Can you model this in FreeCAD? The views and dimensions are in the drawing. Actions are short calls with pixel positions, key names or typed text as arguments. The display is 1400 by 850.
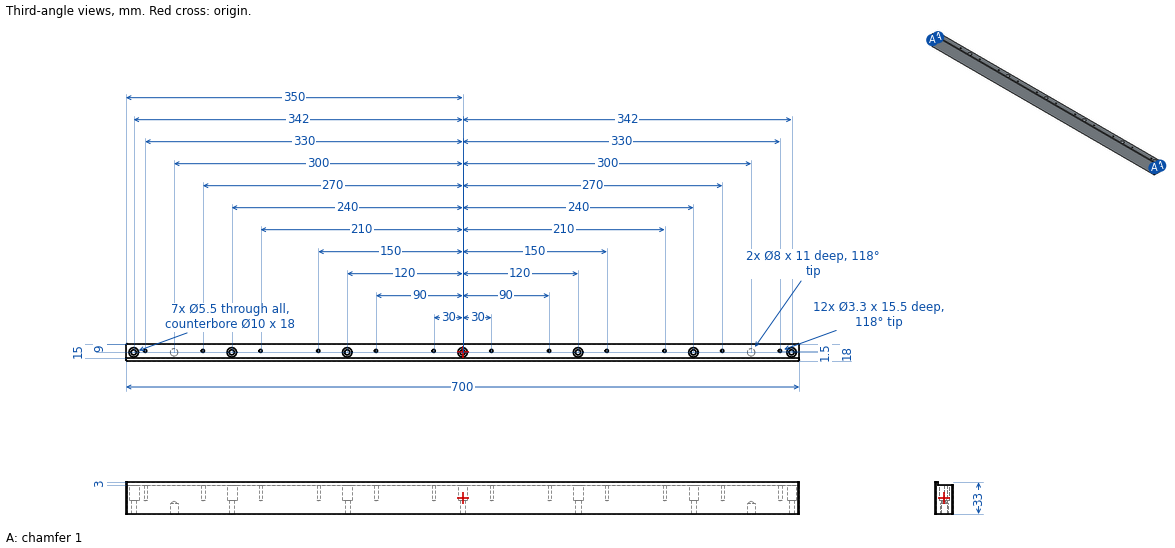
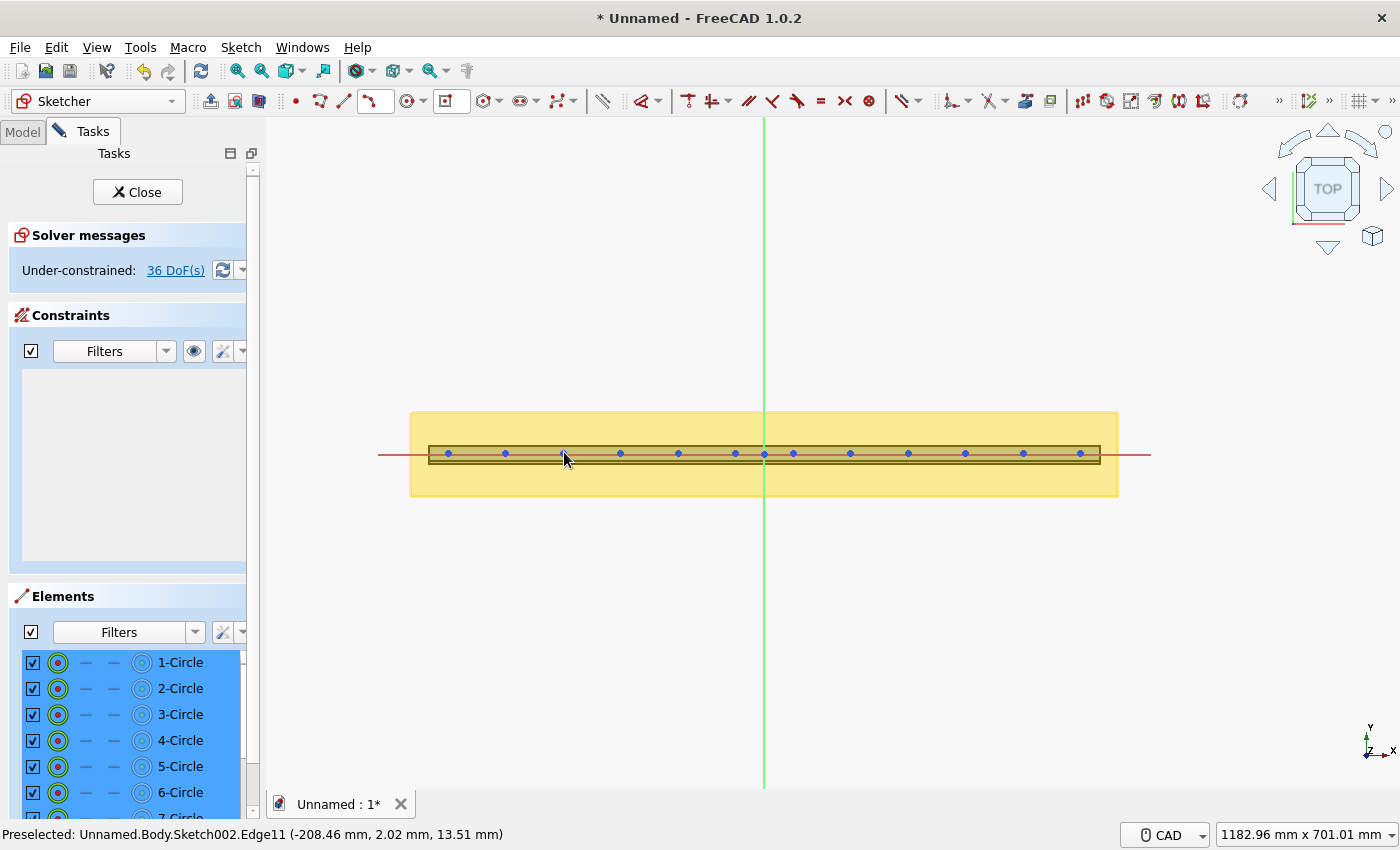
scroll(507, 452, up, 11)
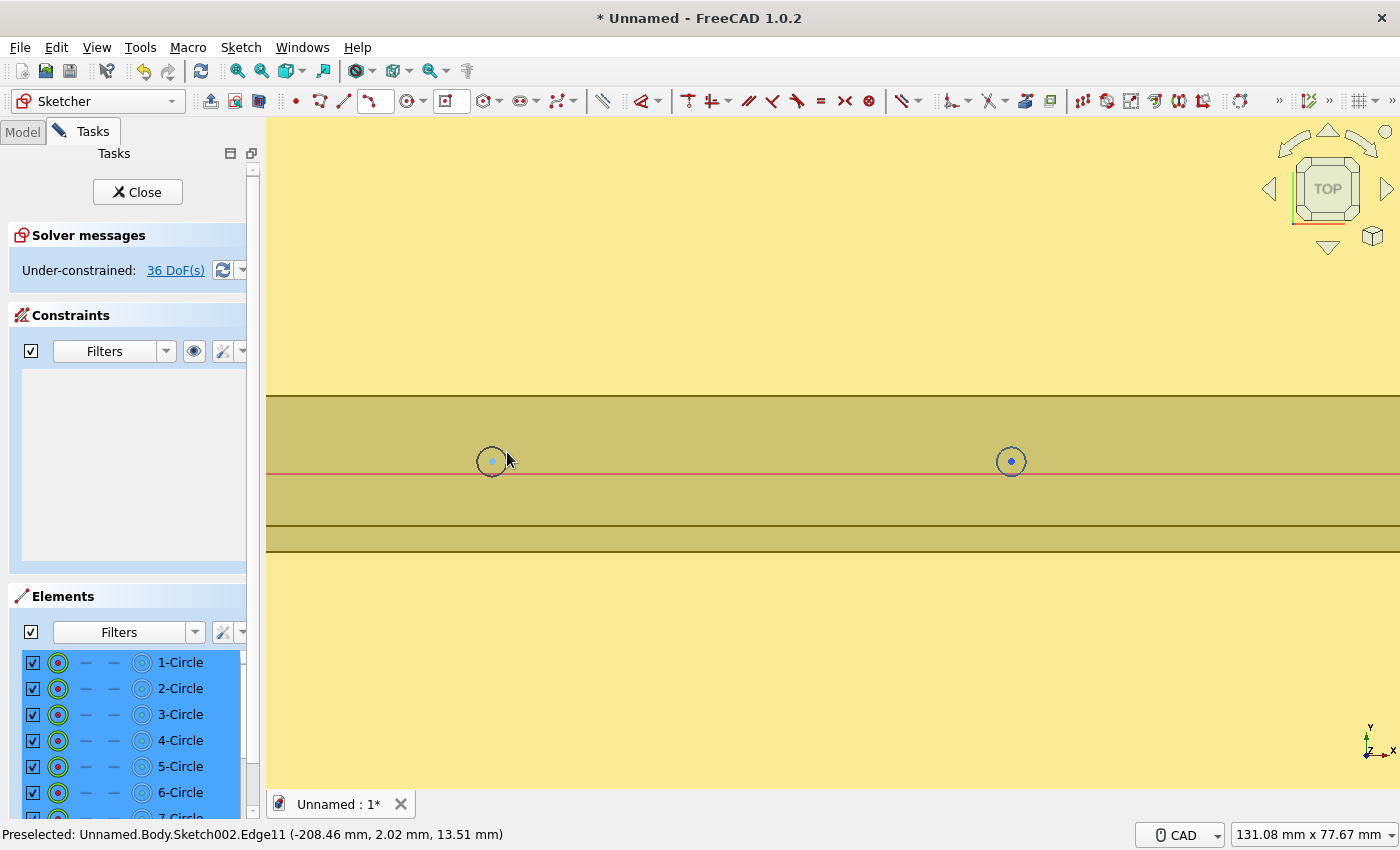
click(502, 451)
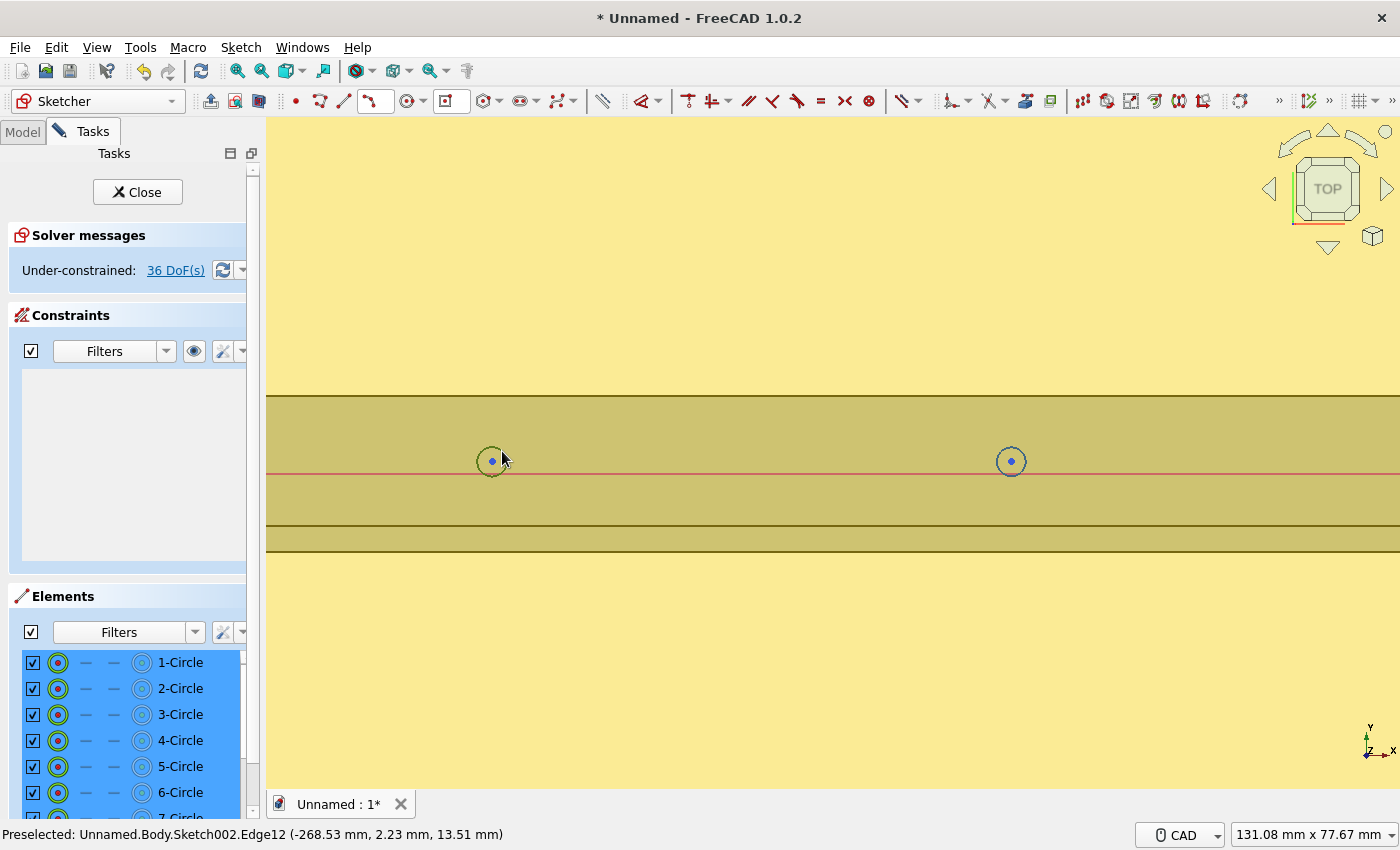
key(e)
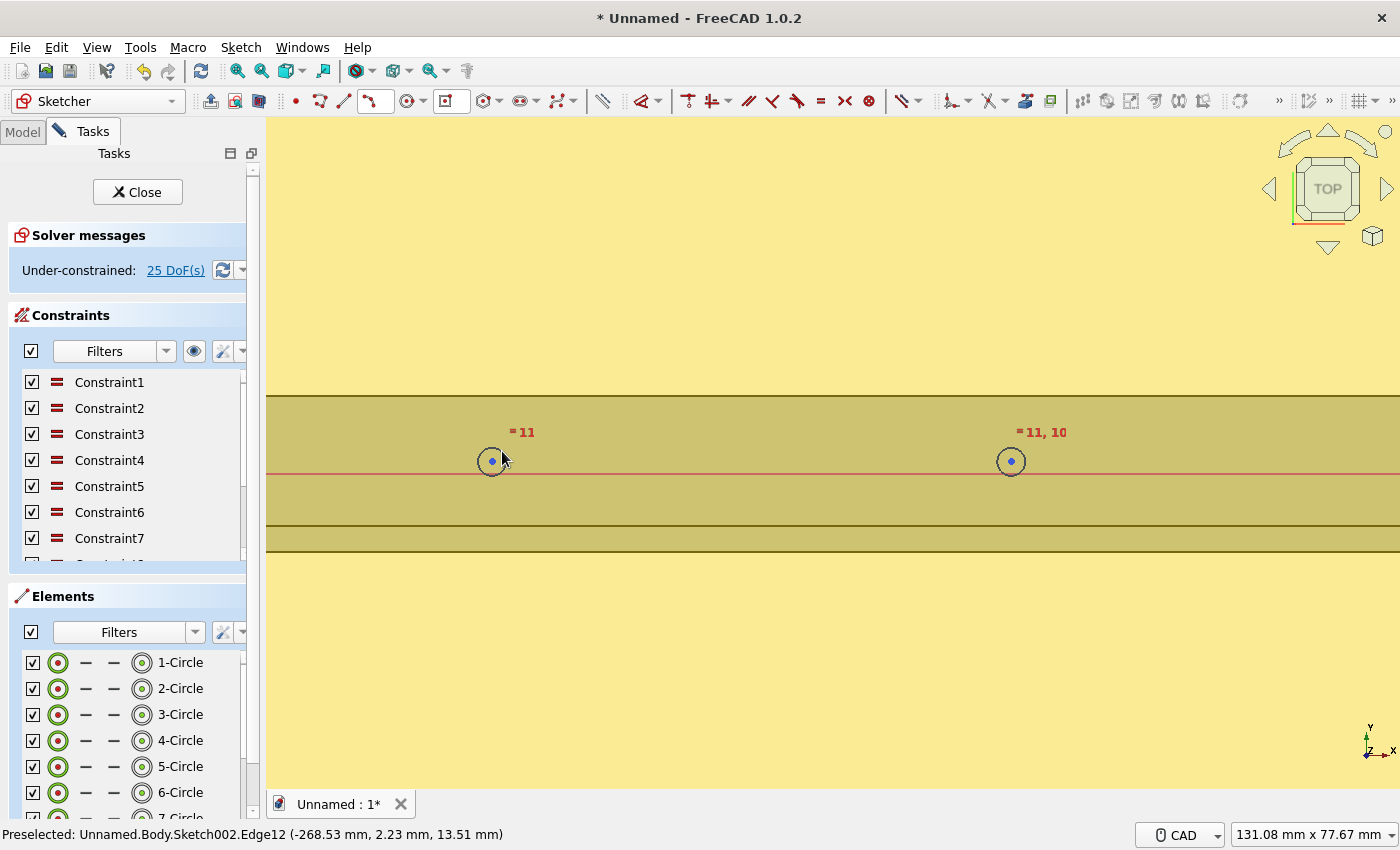
scroll(507, 452, down, 11)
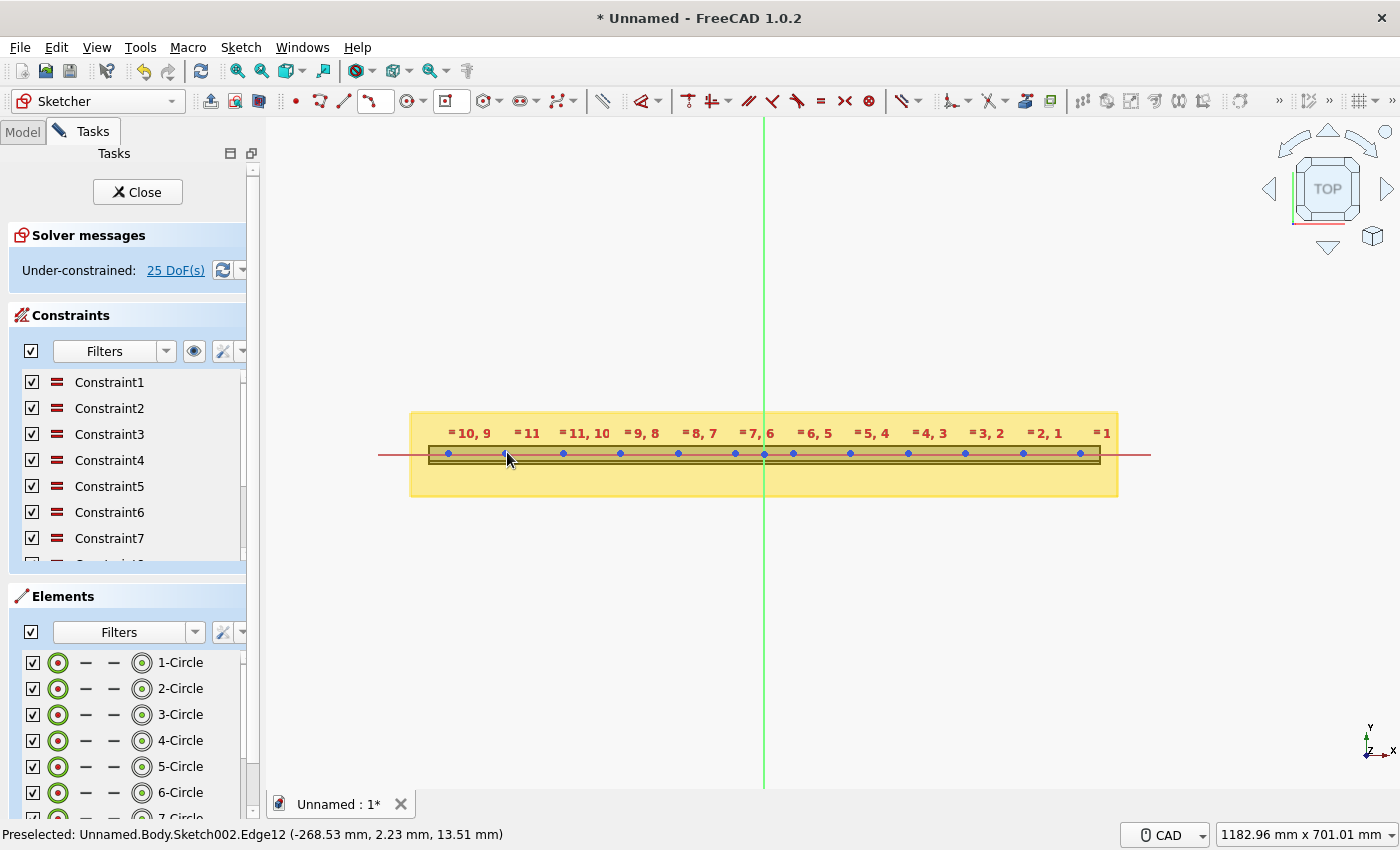
click(1081, 453)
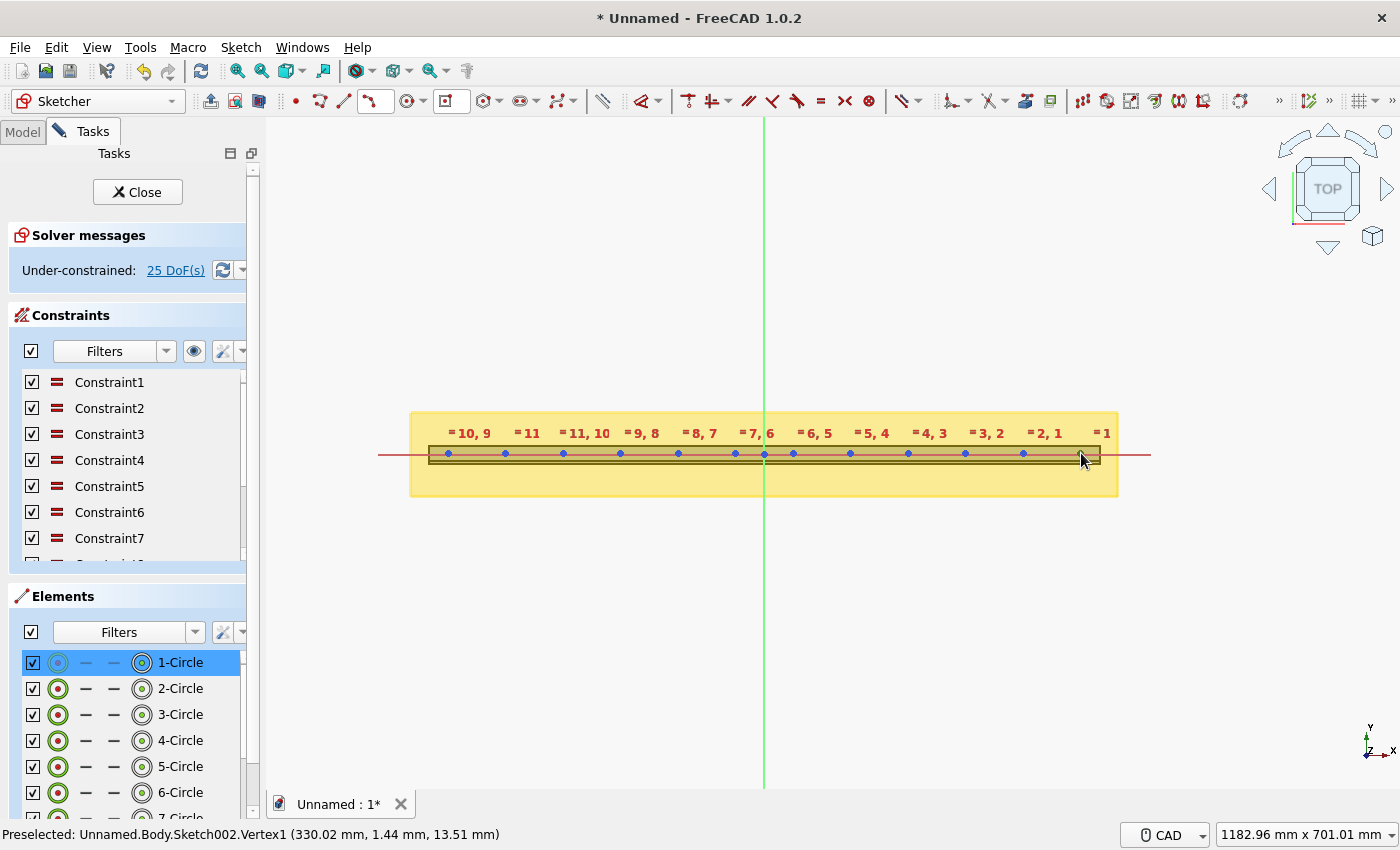
click(1023, 454)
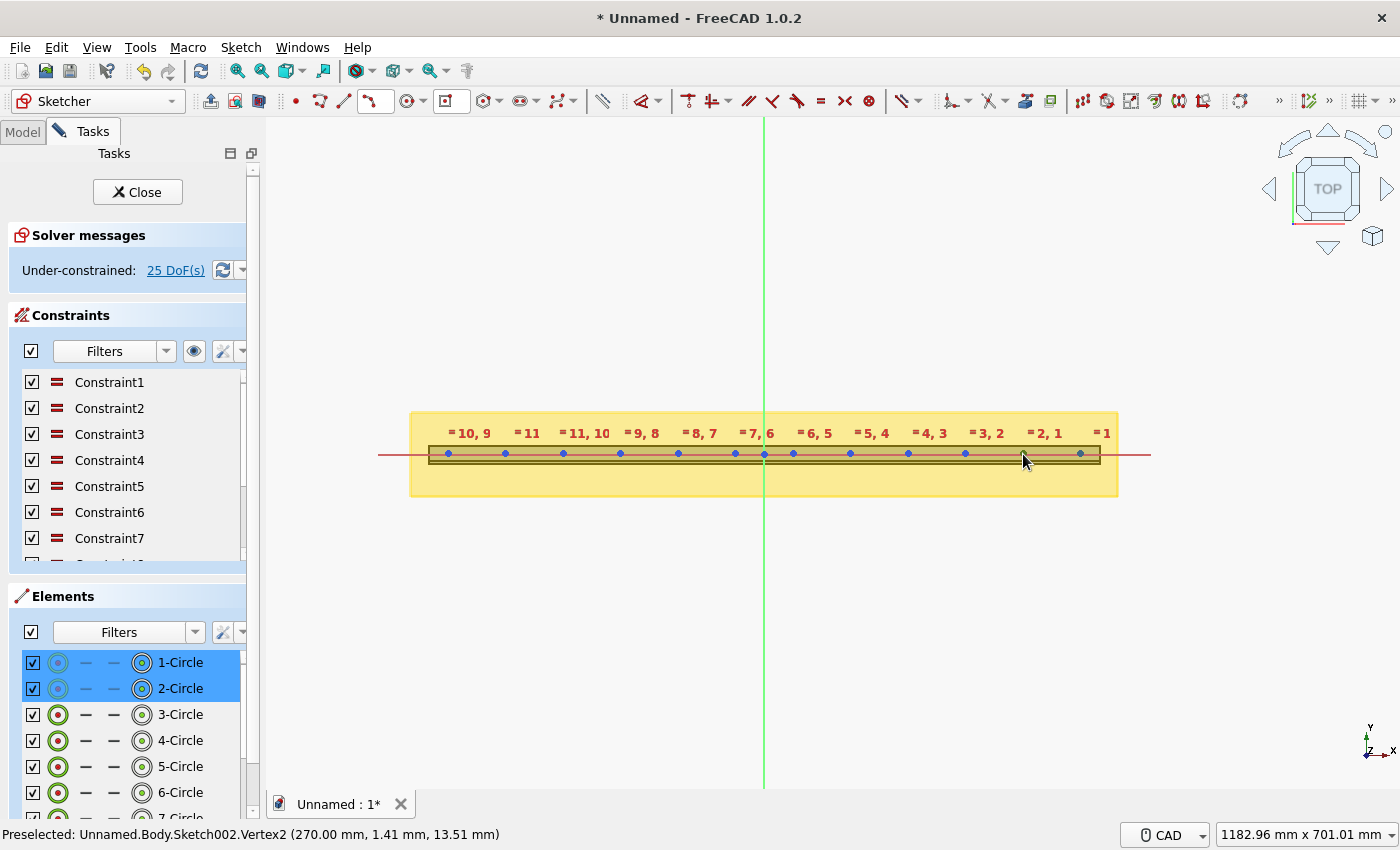
key(h)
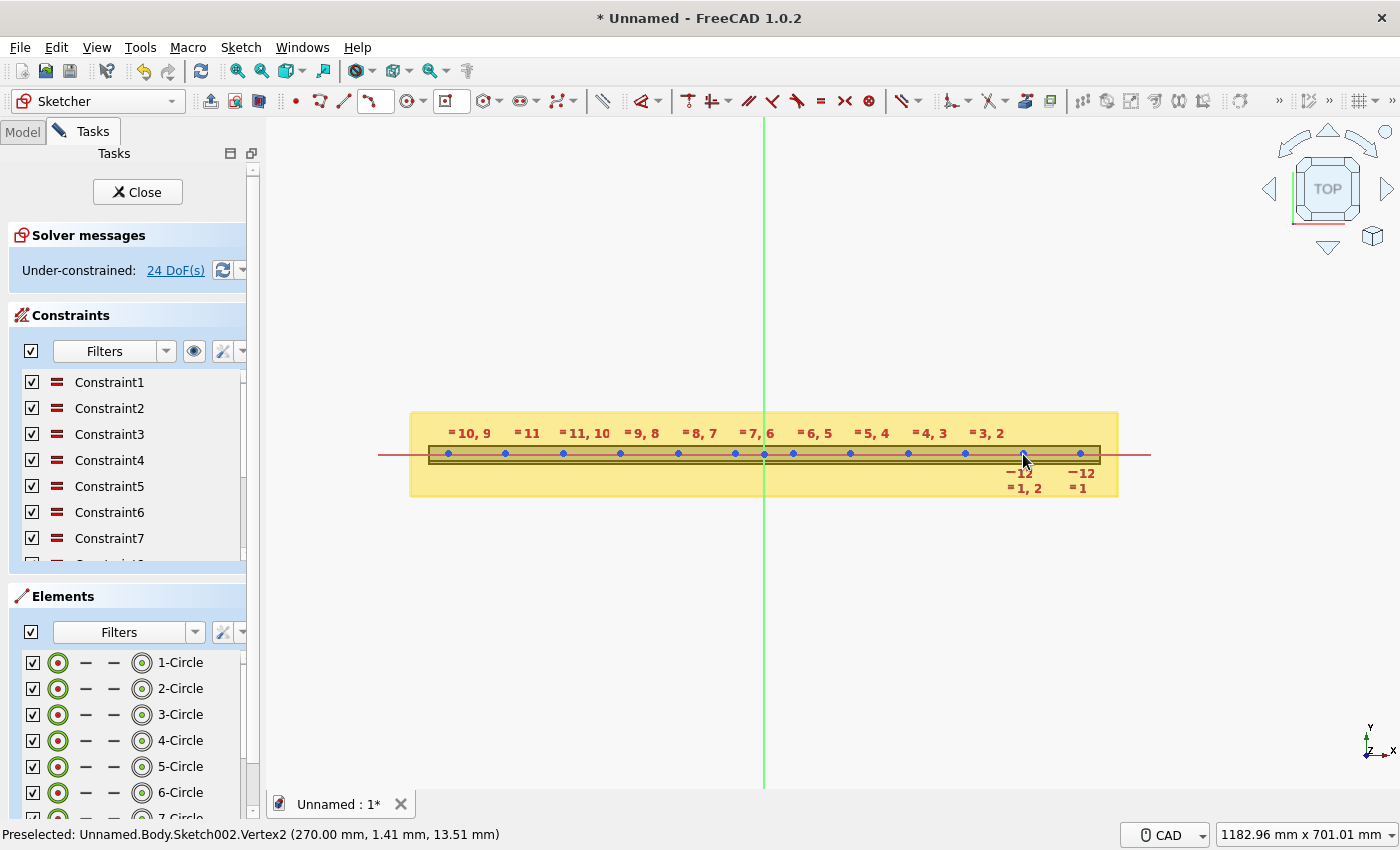
click(1023, 453)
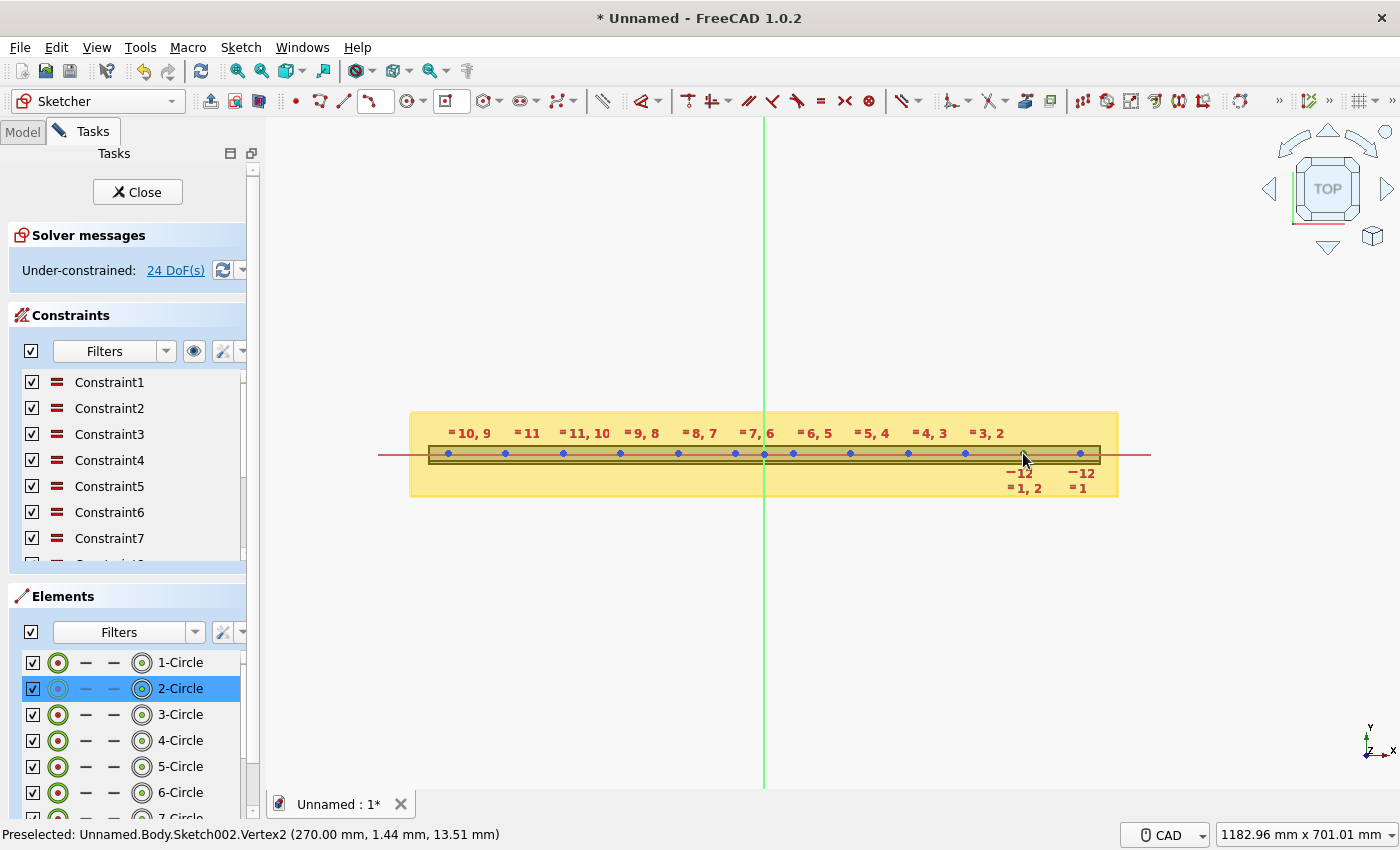
click(966, 454)